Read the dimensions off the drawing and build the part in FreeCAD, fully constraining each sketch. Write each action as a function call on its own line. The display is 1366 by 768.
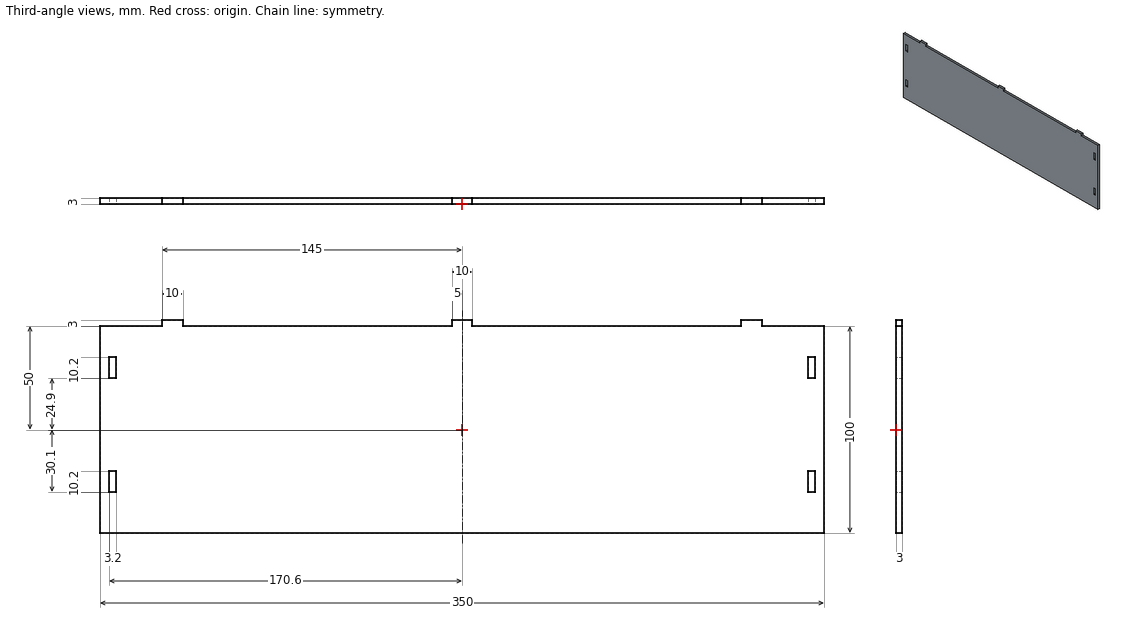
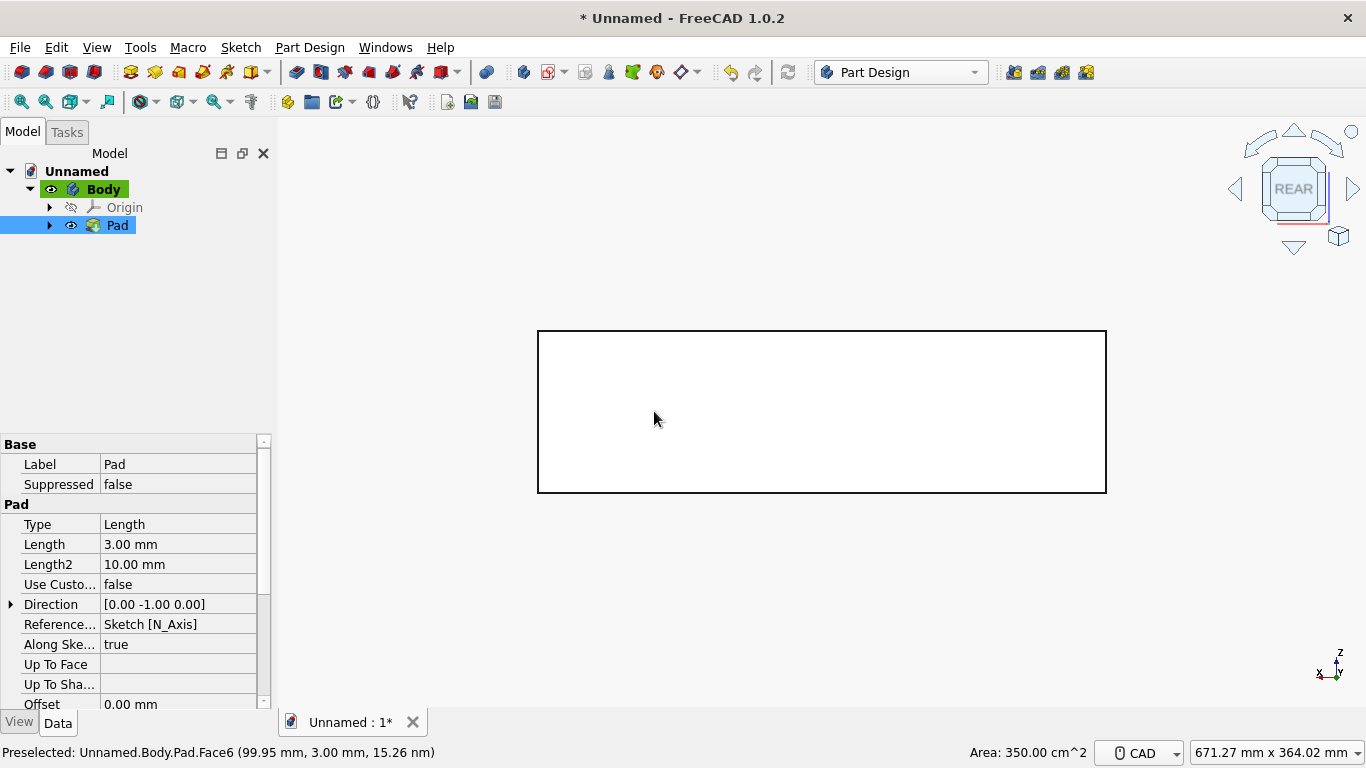
click(548, 72)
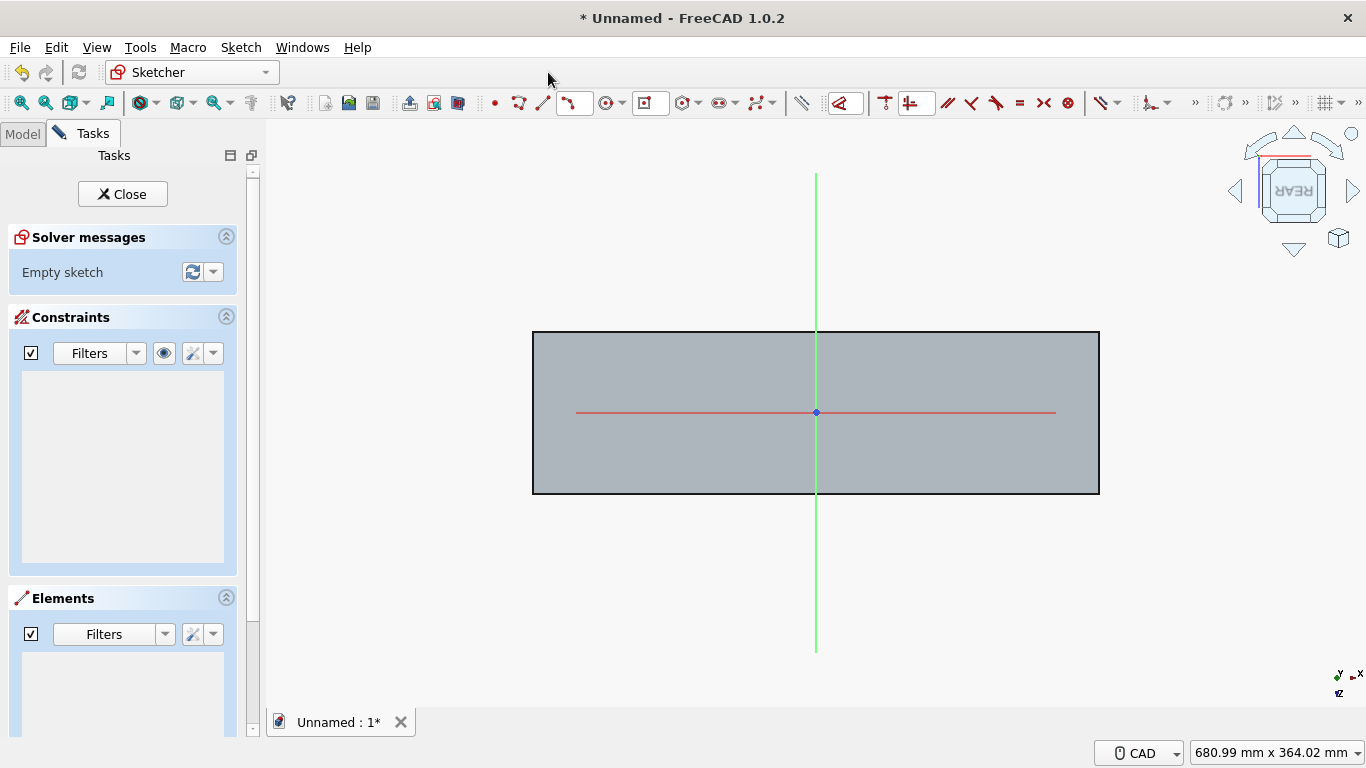
click(664, 104)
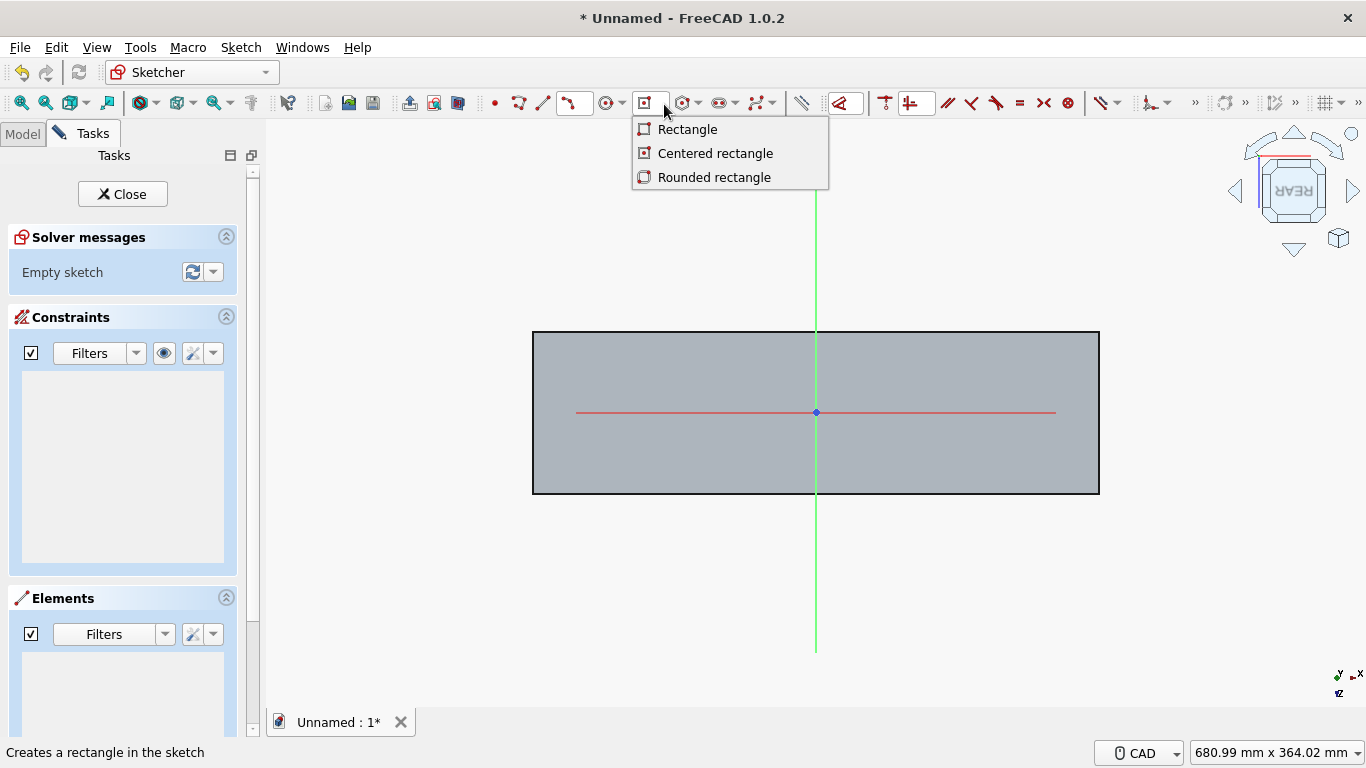
click(730, 129)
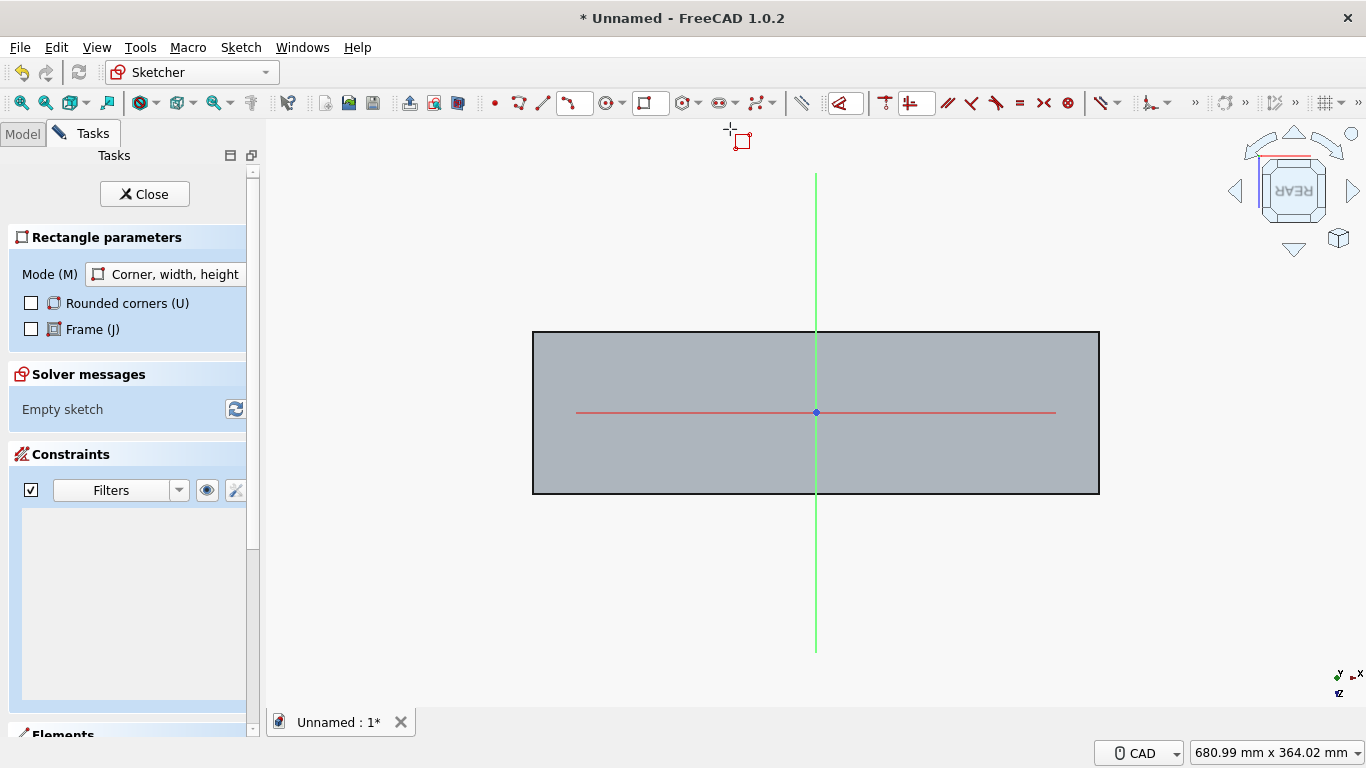
scroll(540, 364, up, 6)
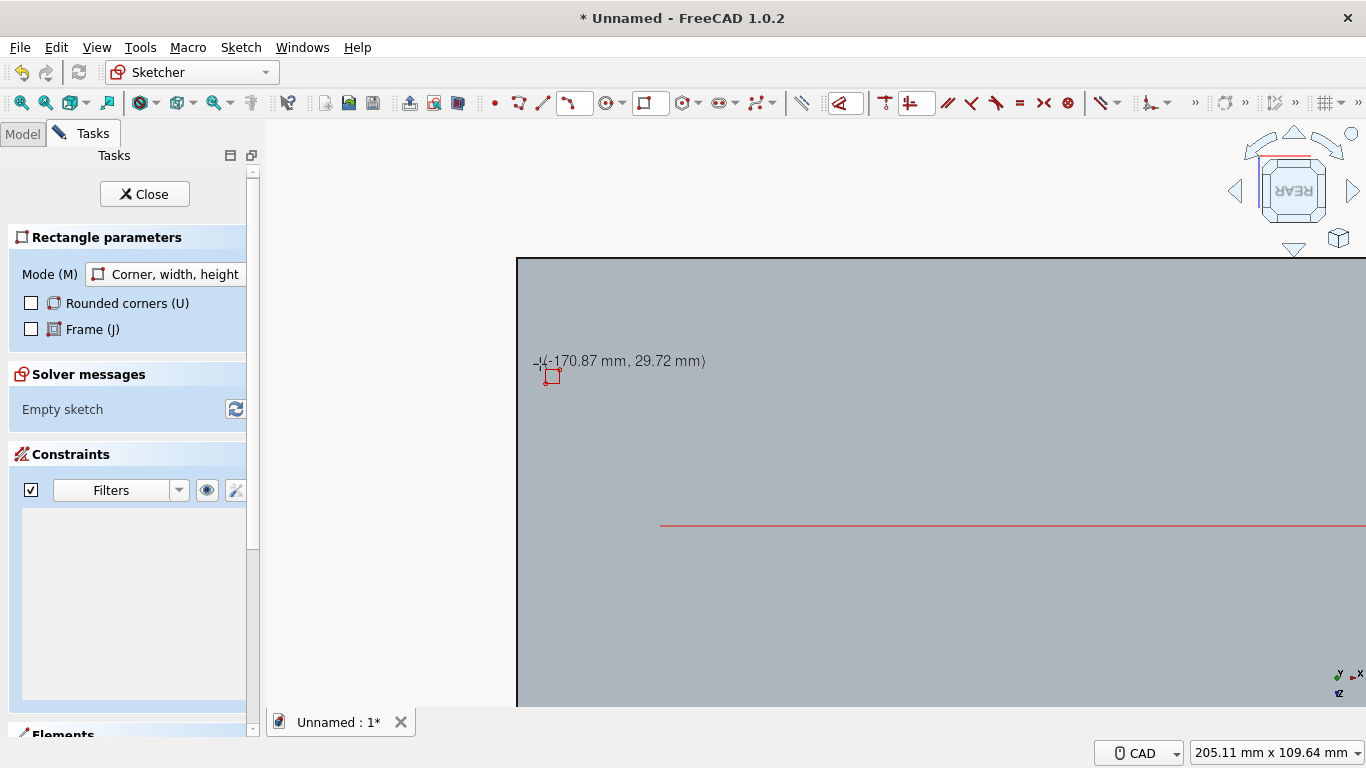
click(541, 364)
click(558, 419)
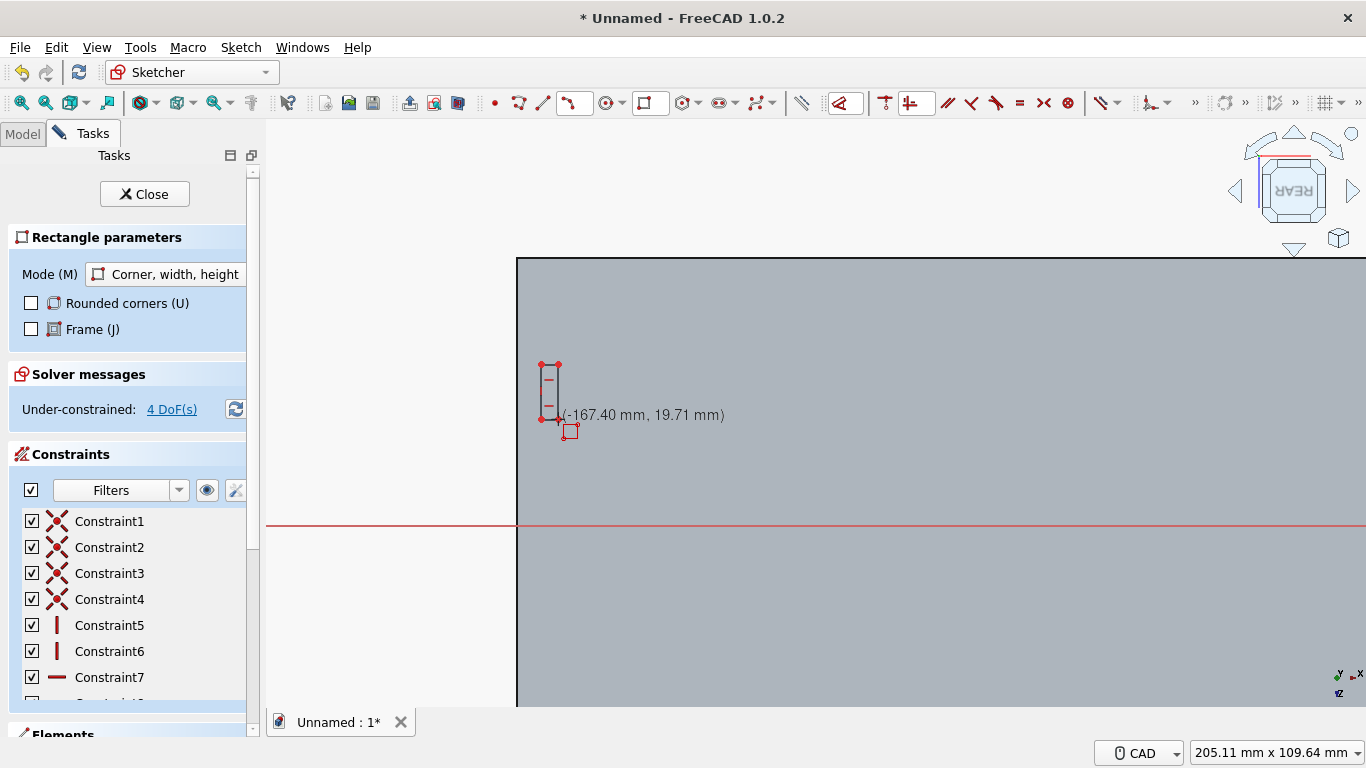
click(541, 659)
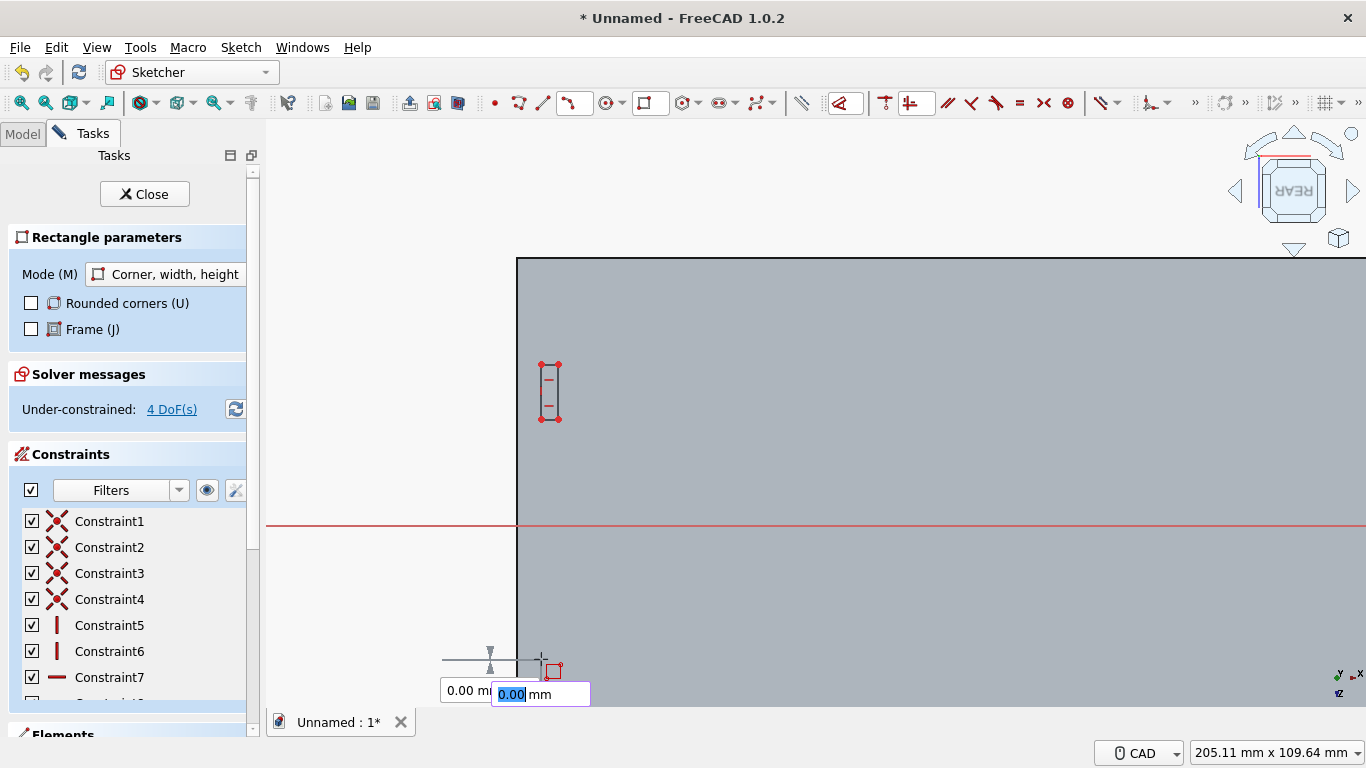
scroll(335, 340, down, 5)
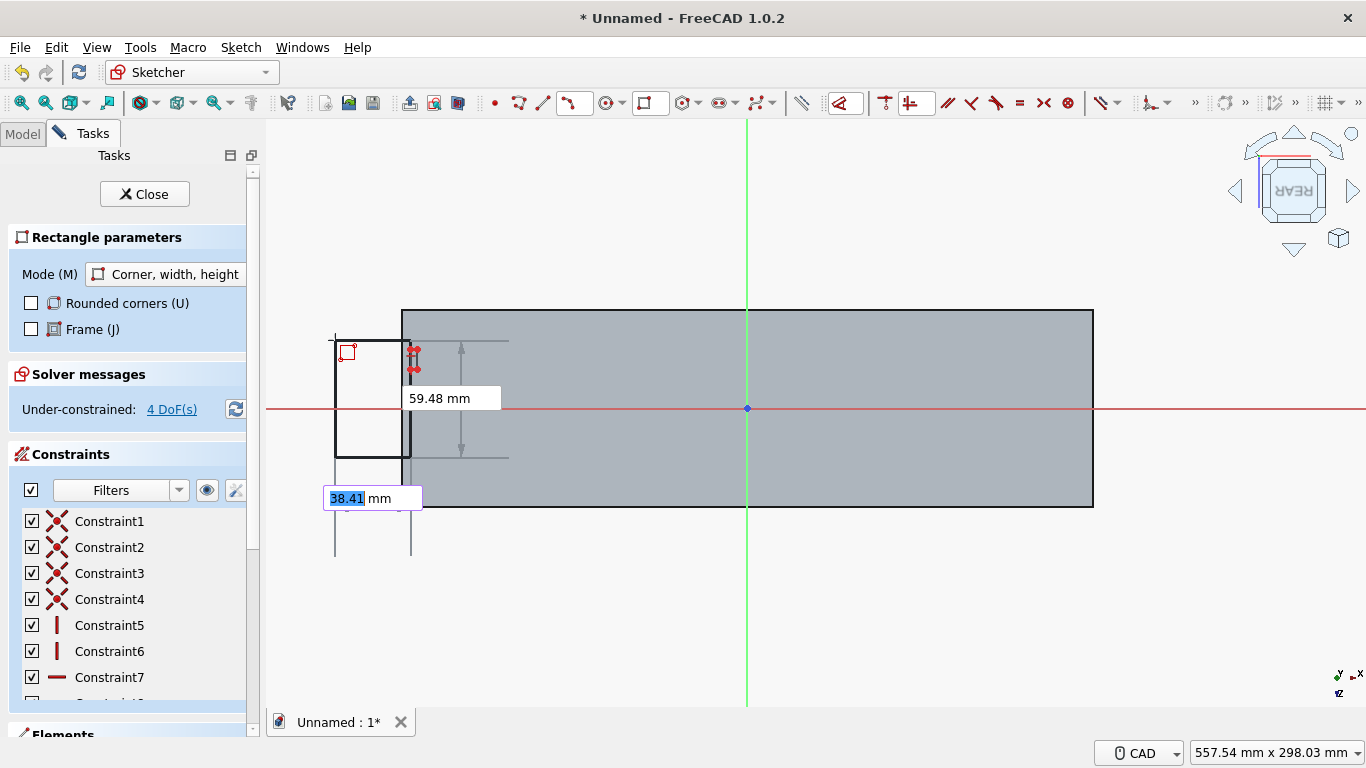
click(417, 478)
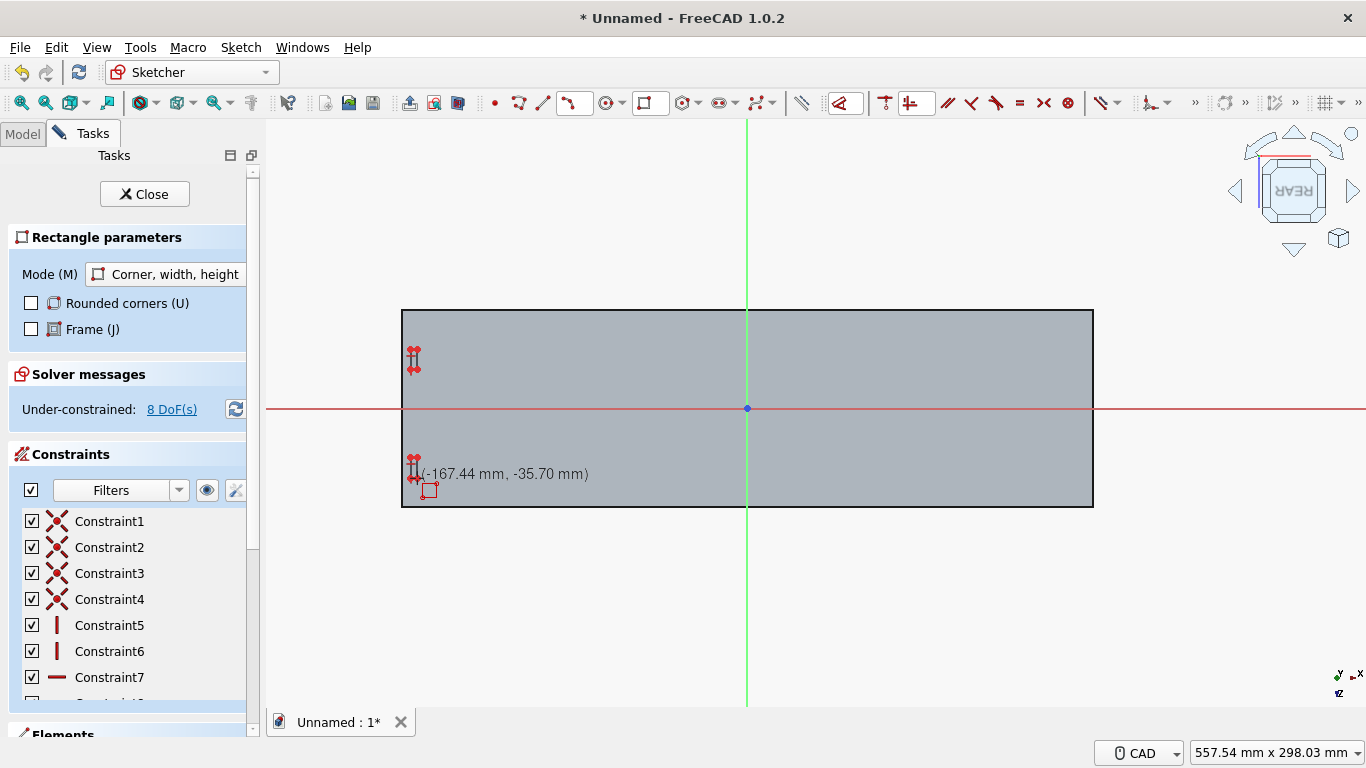
scroll(1078, 458, up, 5)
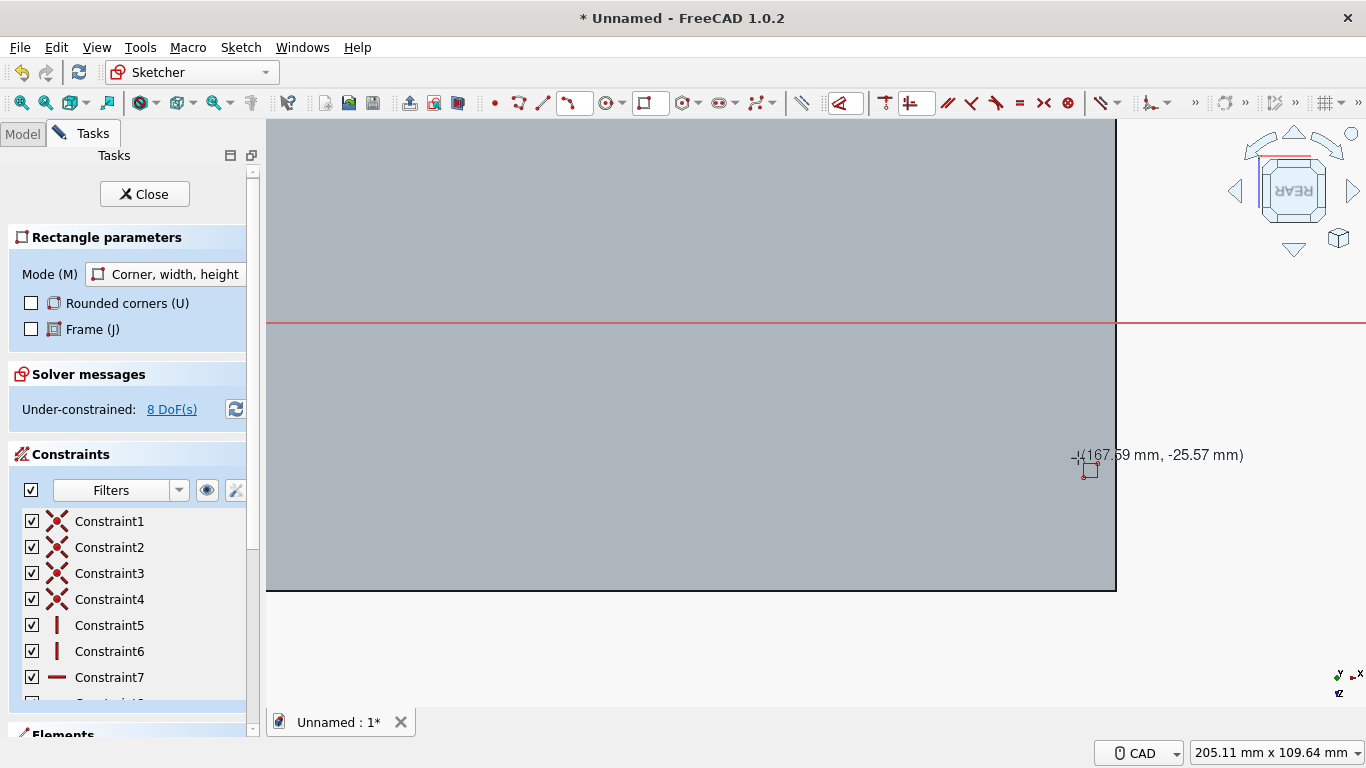
click(1076, 456)
click(1093, 511)